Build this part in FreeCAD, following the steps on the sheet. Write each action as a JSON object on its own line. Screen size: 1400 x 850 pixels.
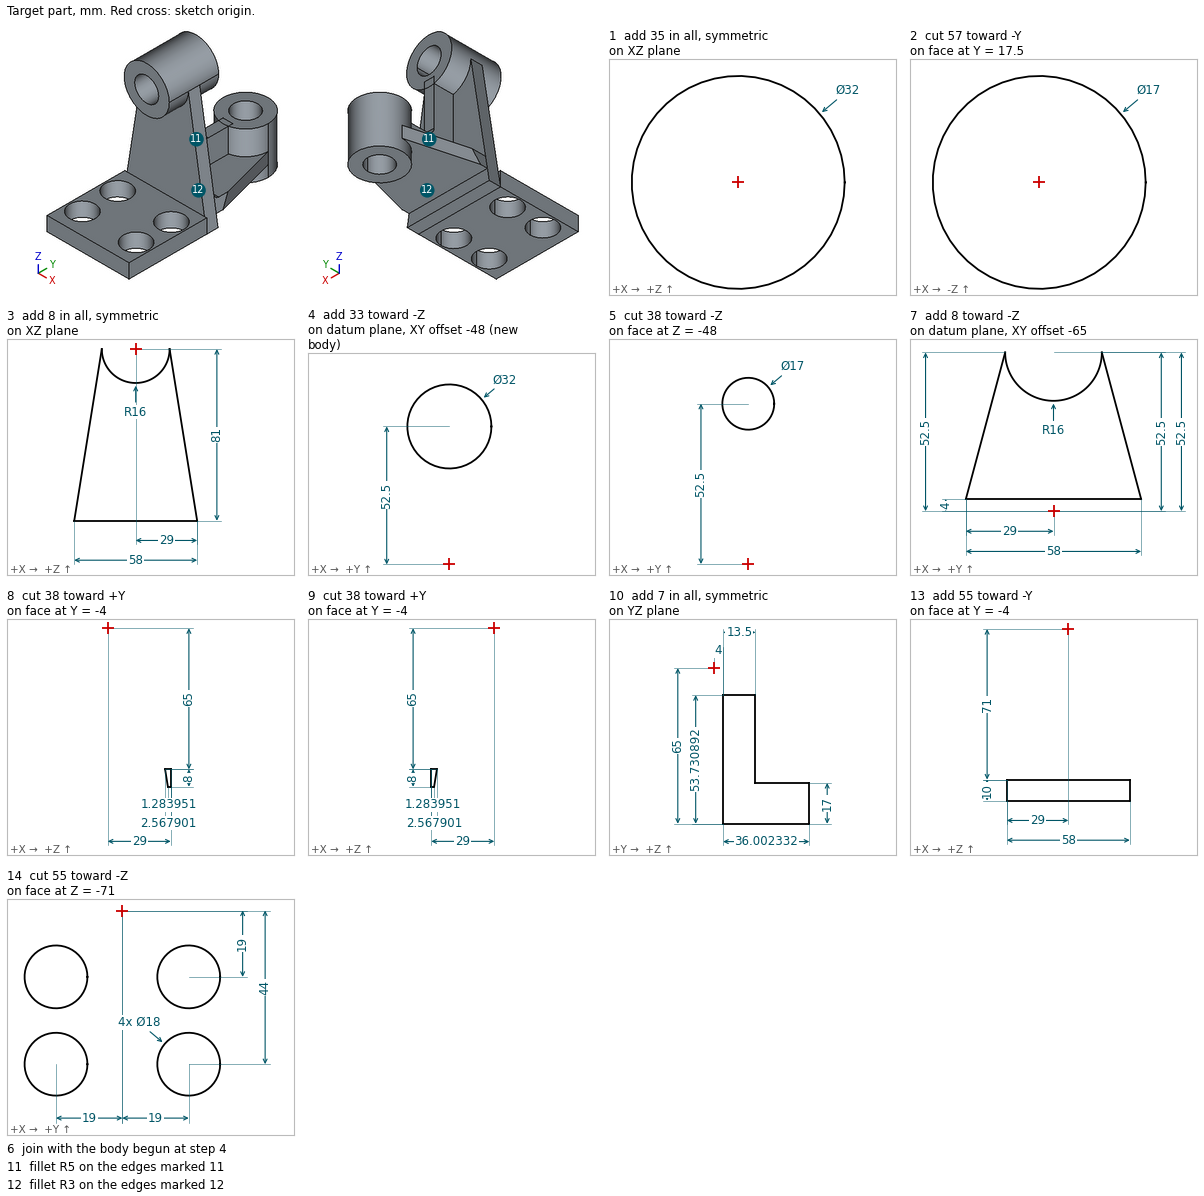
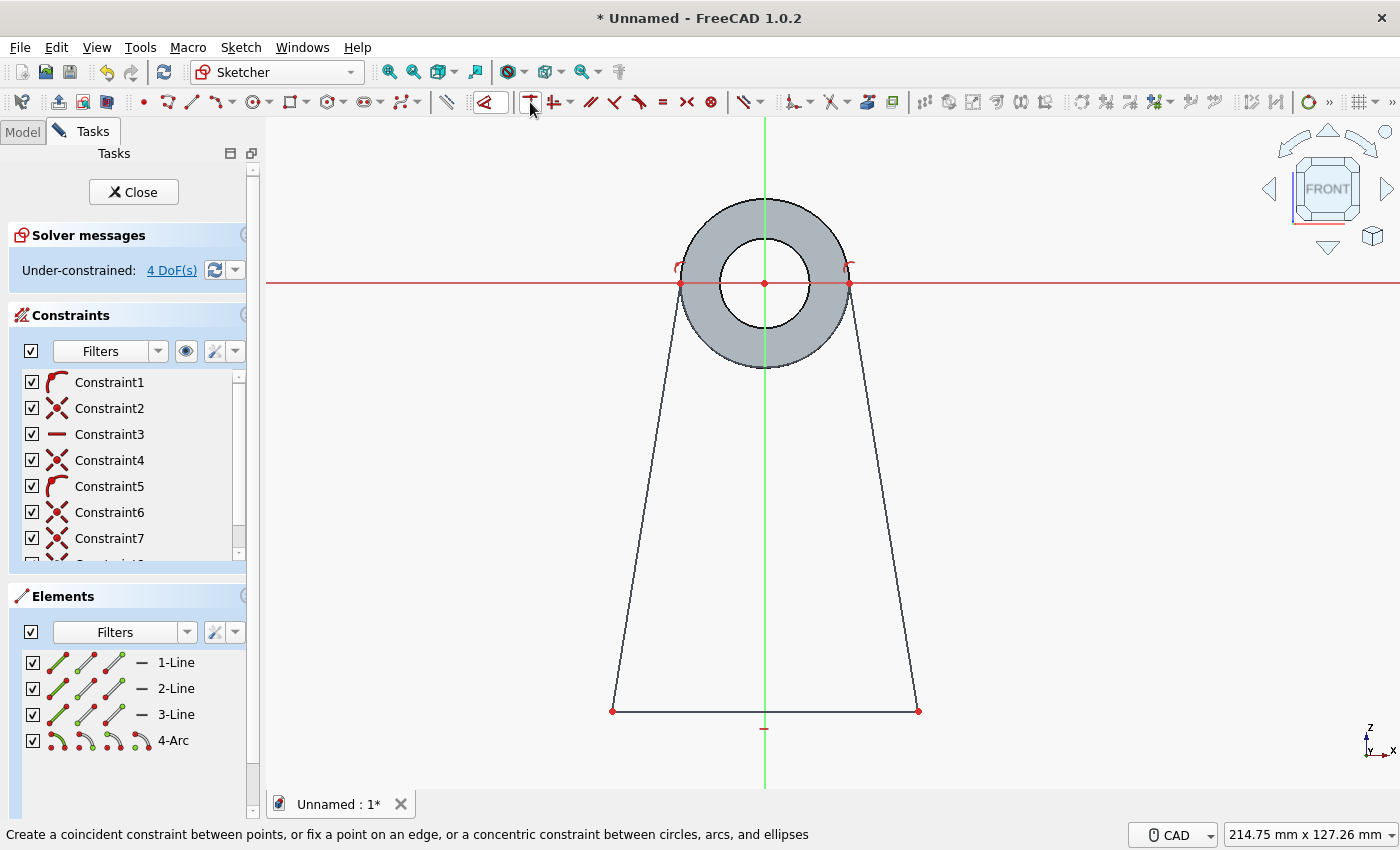
{"action": "key", "text": "d"}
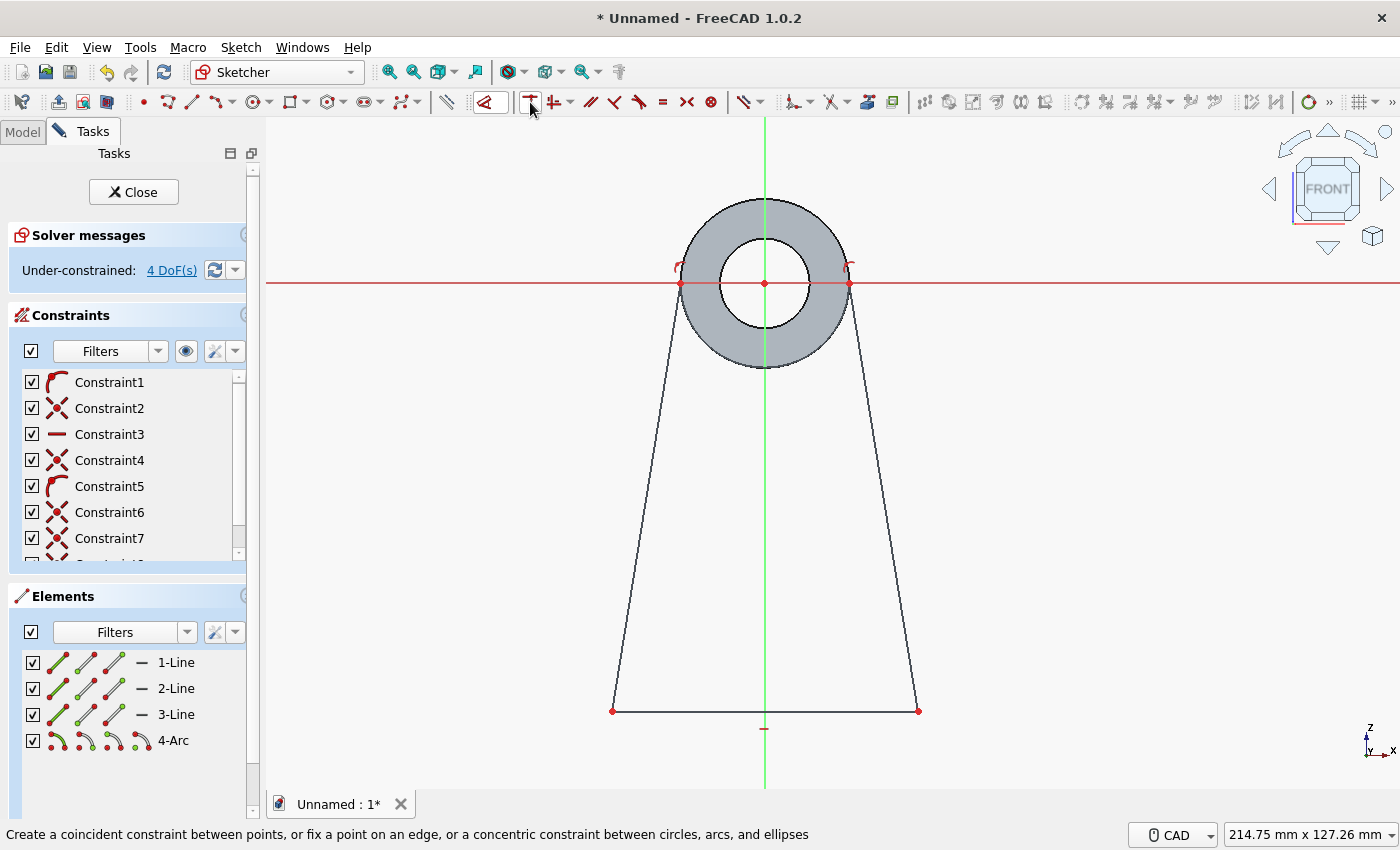
{"action": "left_click", "coordinate": [715, 351]}
{"action": "left_click", "coordinate": [696, 377]}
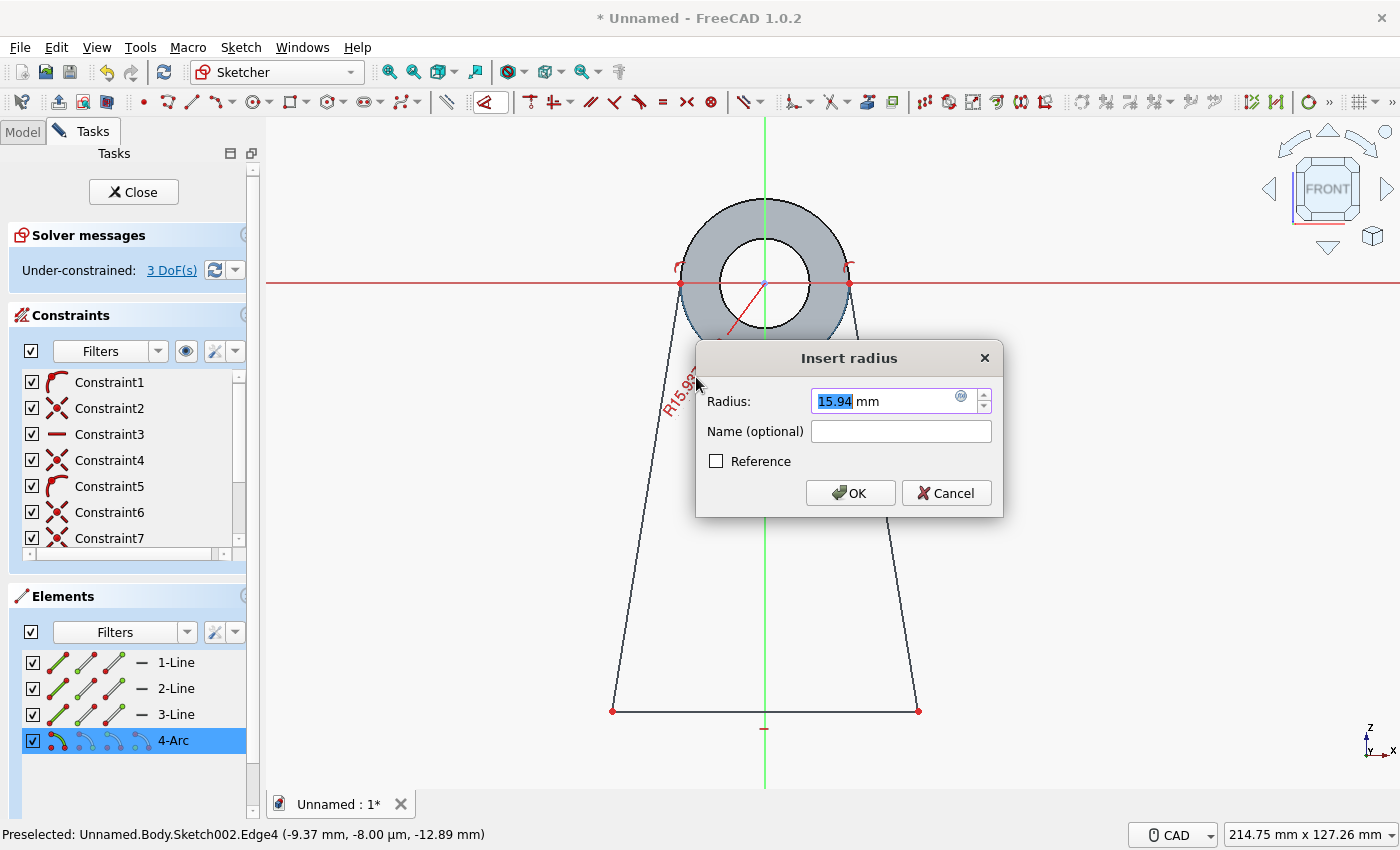
{"action": "type", "text": "16"}
{"action": "key", "text": "Return"}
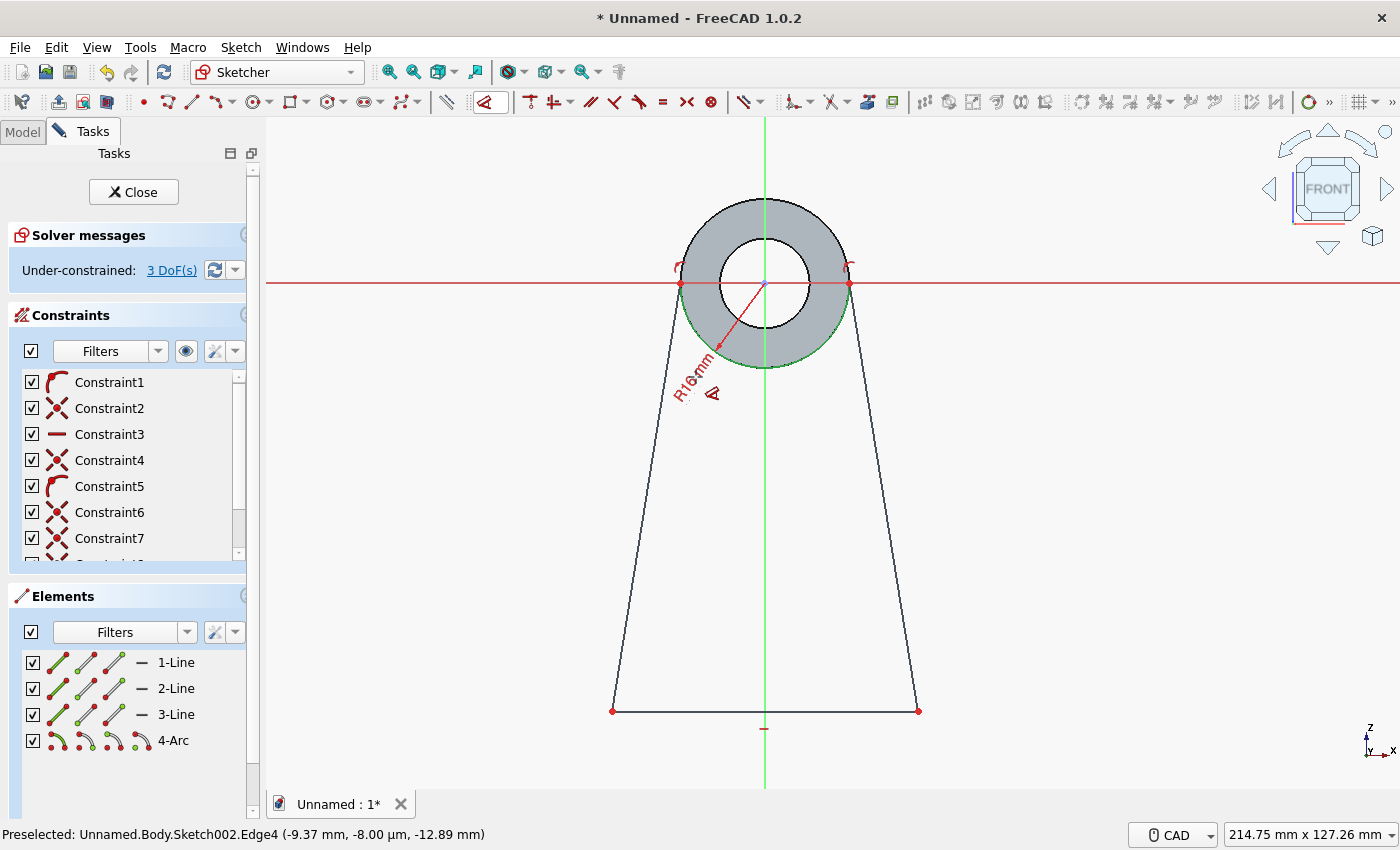
{"action": "left_click", "coordinate": [826, 712]}
{"action": "left_click", "coordinate": [695, 746]}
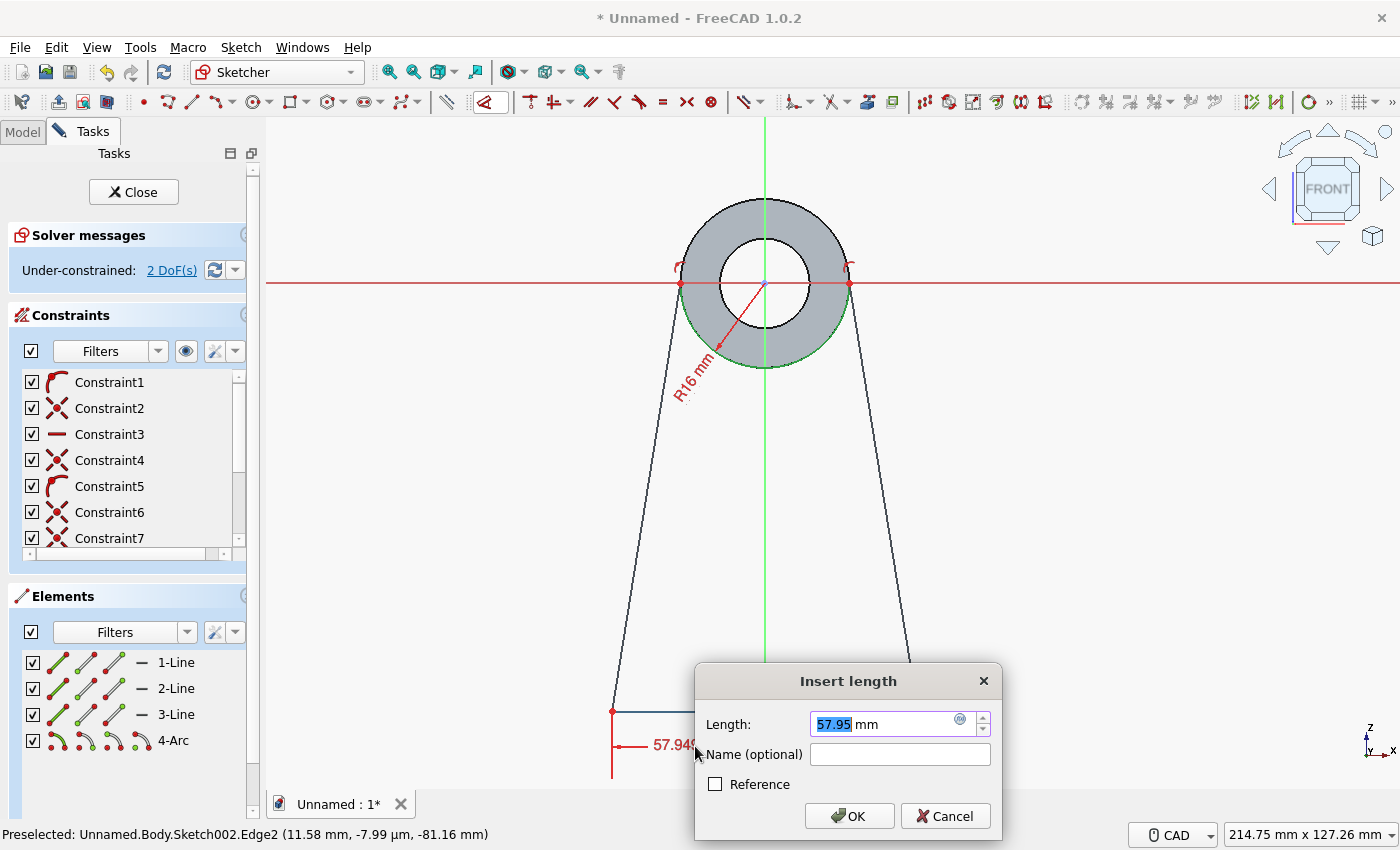
{"action": "type", "text": "58"}
{"action": "key", "text": "Return"}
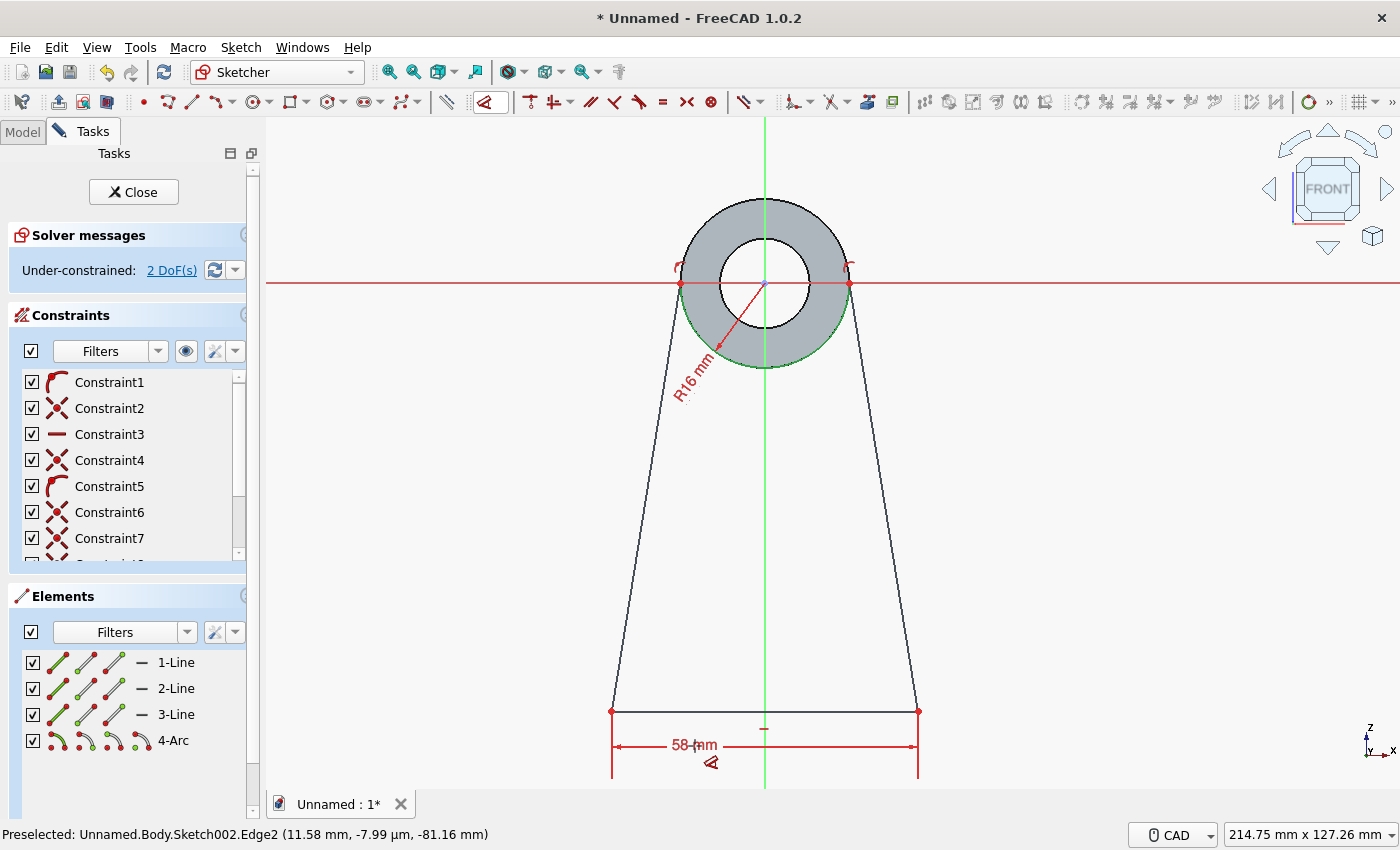
{"action": "left_click", "coordinate": [918, 712]}
{"action": "left_click", "coordinate": [841, 746]}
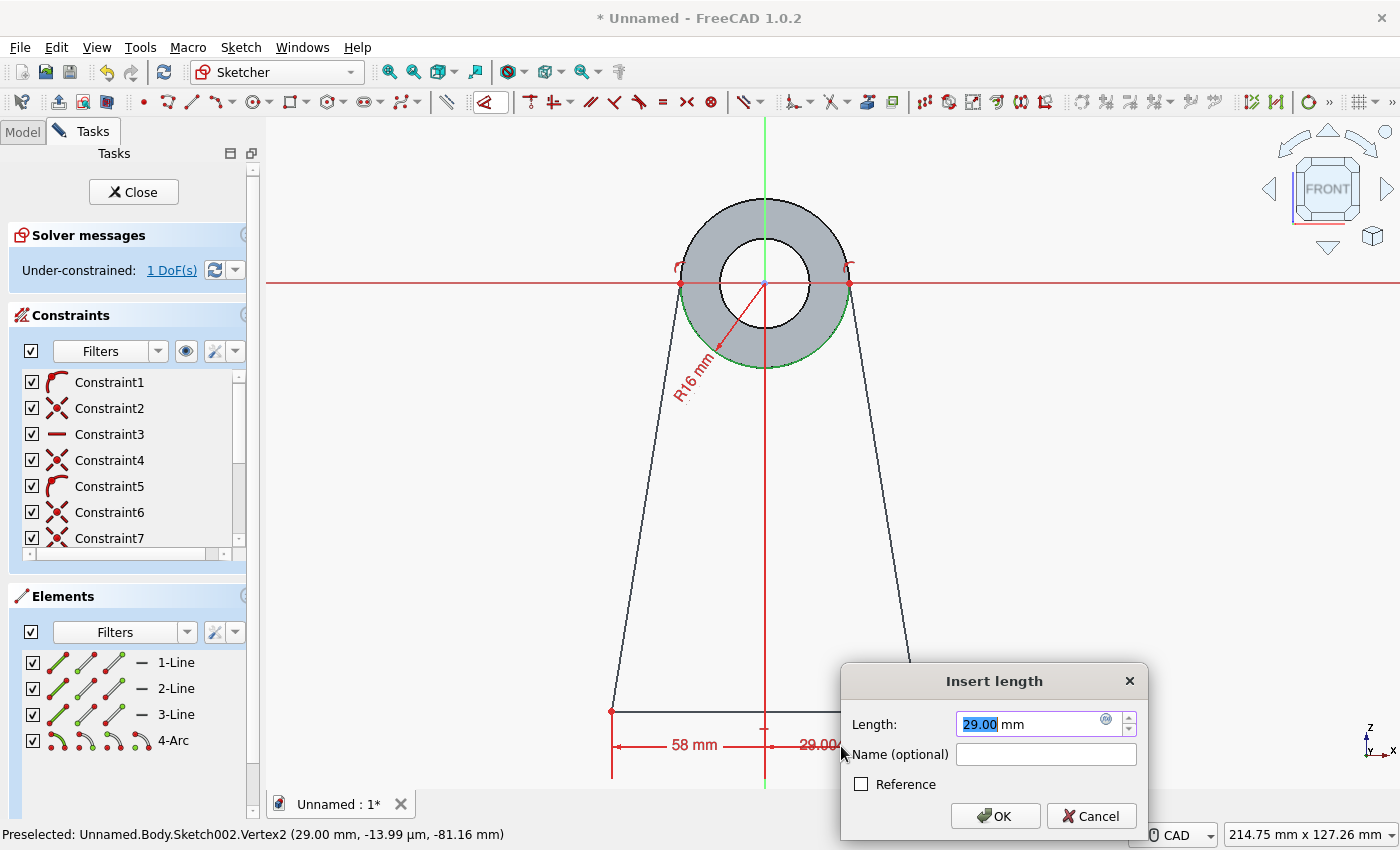
{"action": "type", "text": "29"}
{"action": "key", "text": "Return"}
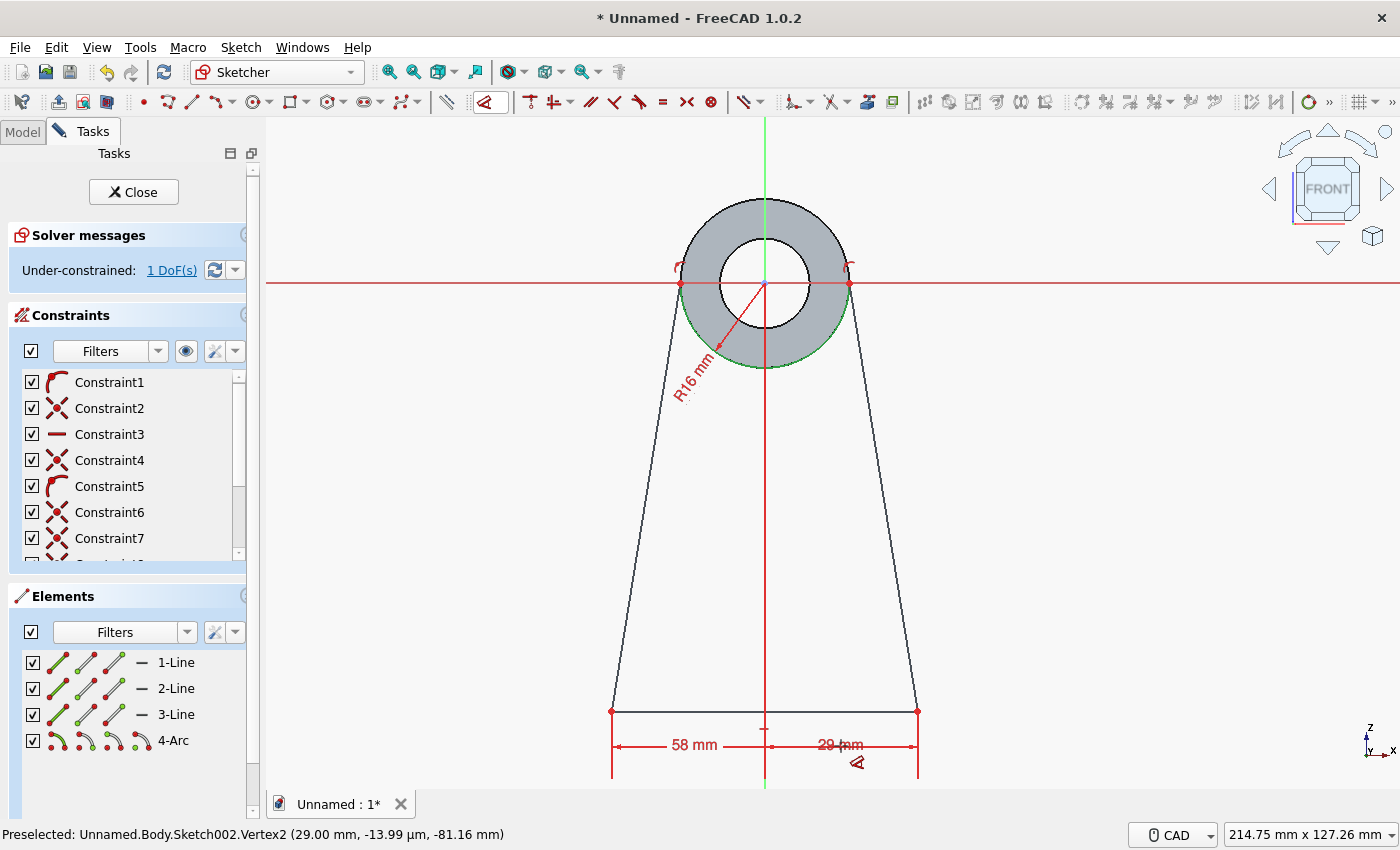
{"action": "left_click", "coordinate": [918, 712]}
{"action": "left_click", "coordinate": [952, 498]}